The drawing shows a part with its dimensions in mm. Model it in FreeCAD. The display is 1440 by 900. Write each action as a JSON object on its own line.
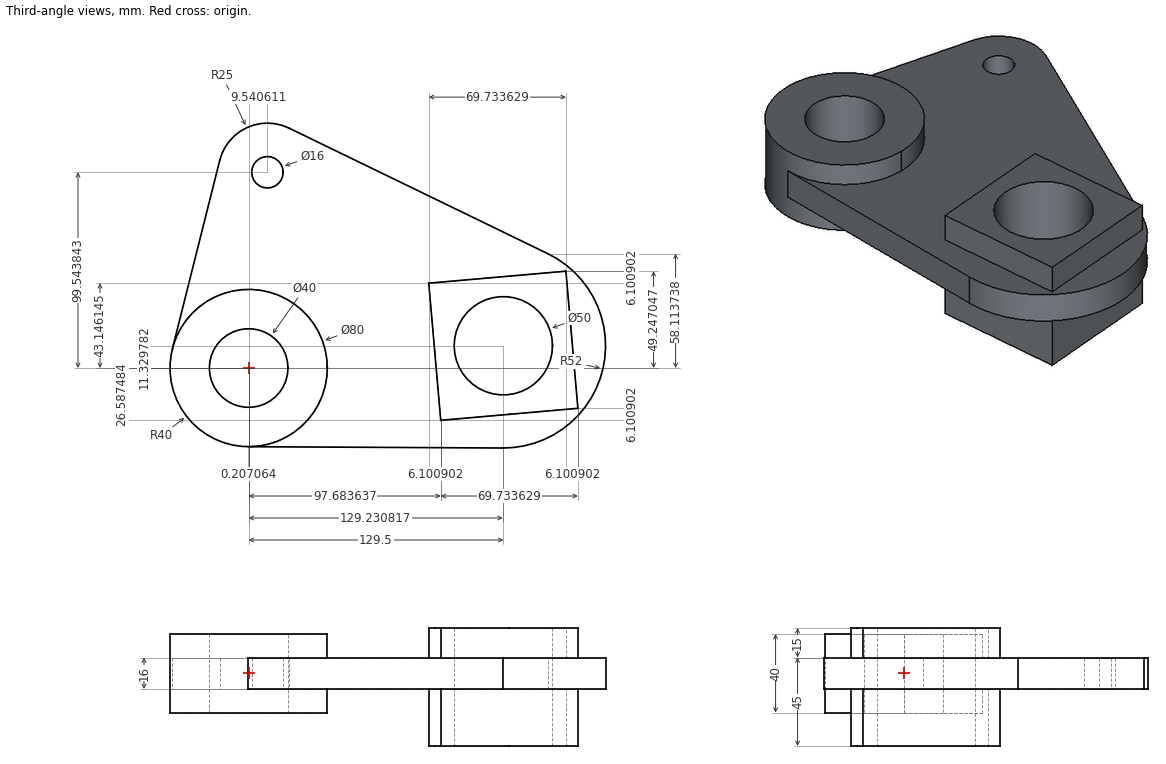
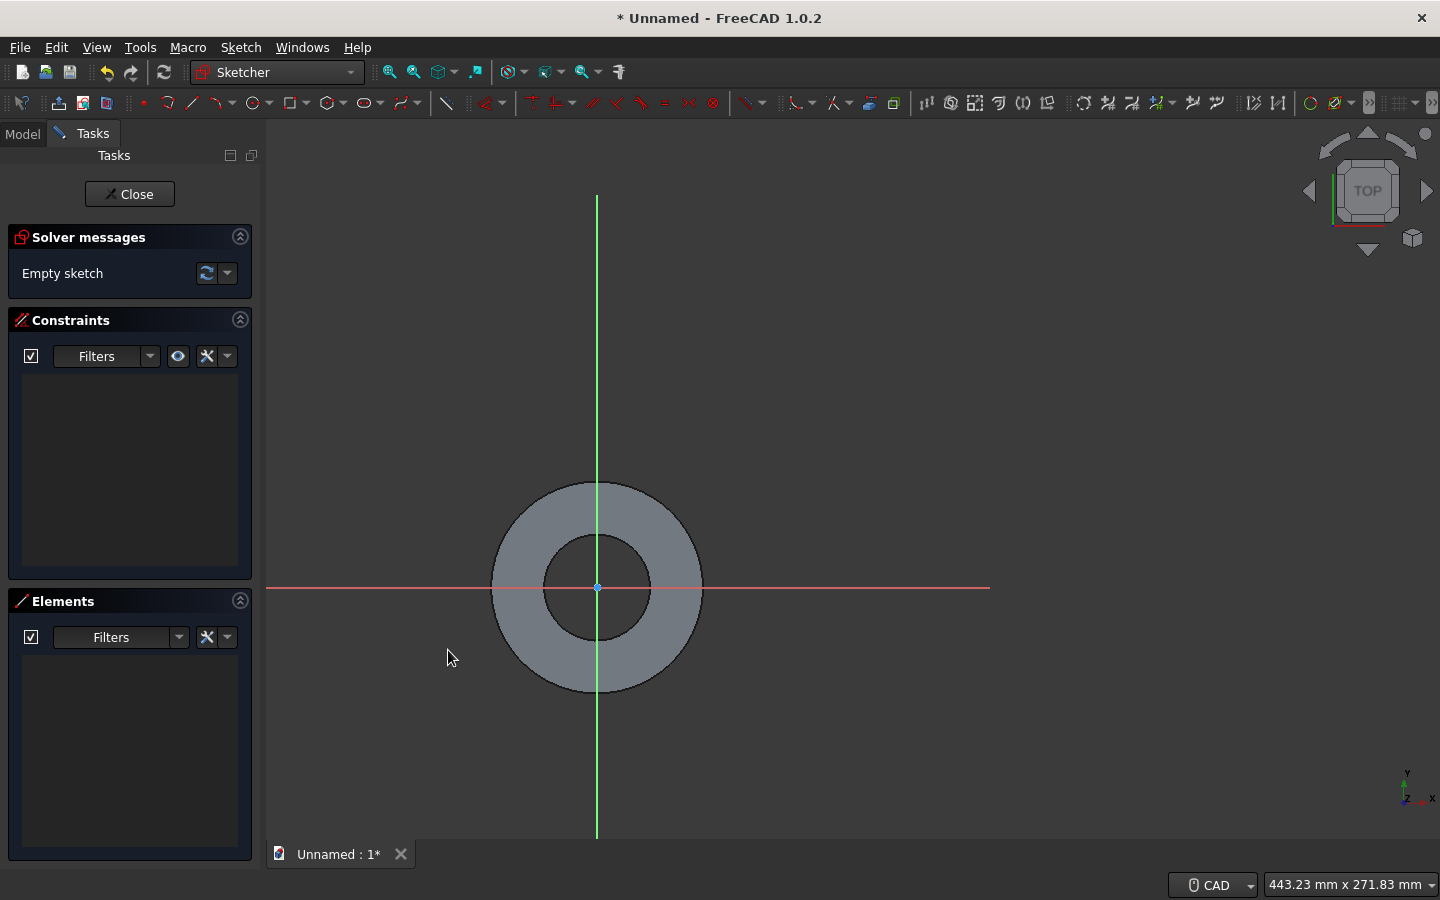
{"action": "key", "text": "g l"}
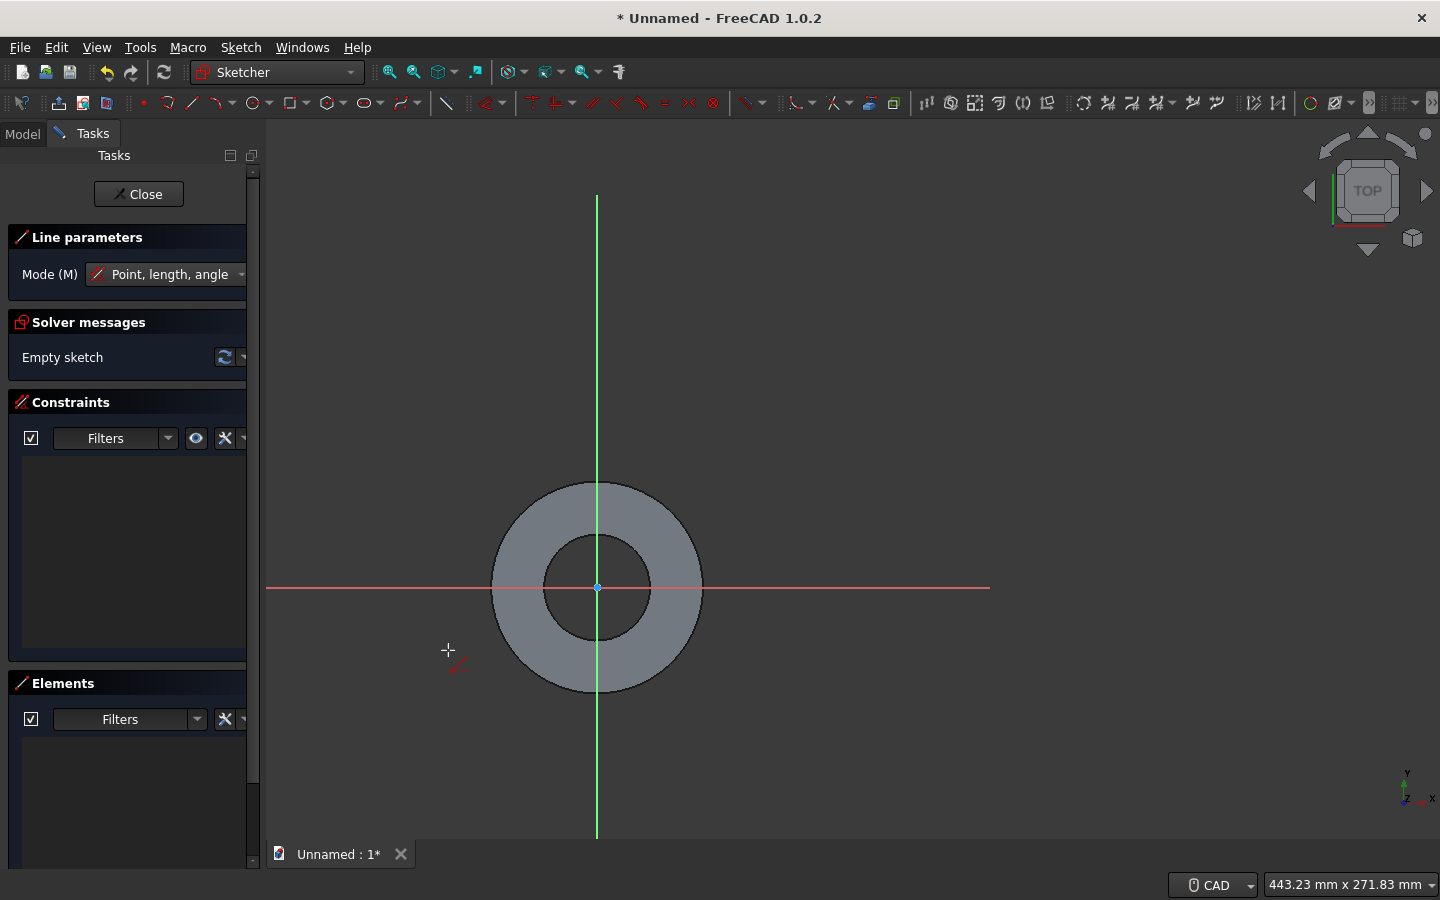
{"action": "scroll", "coordinate": [597, 694], "scroll_direction": "up", "scroll_amount": 17}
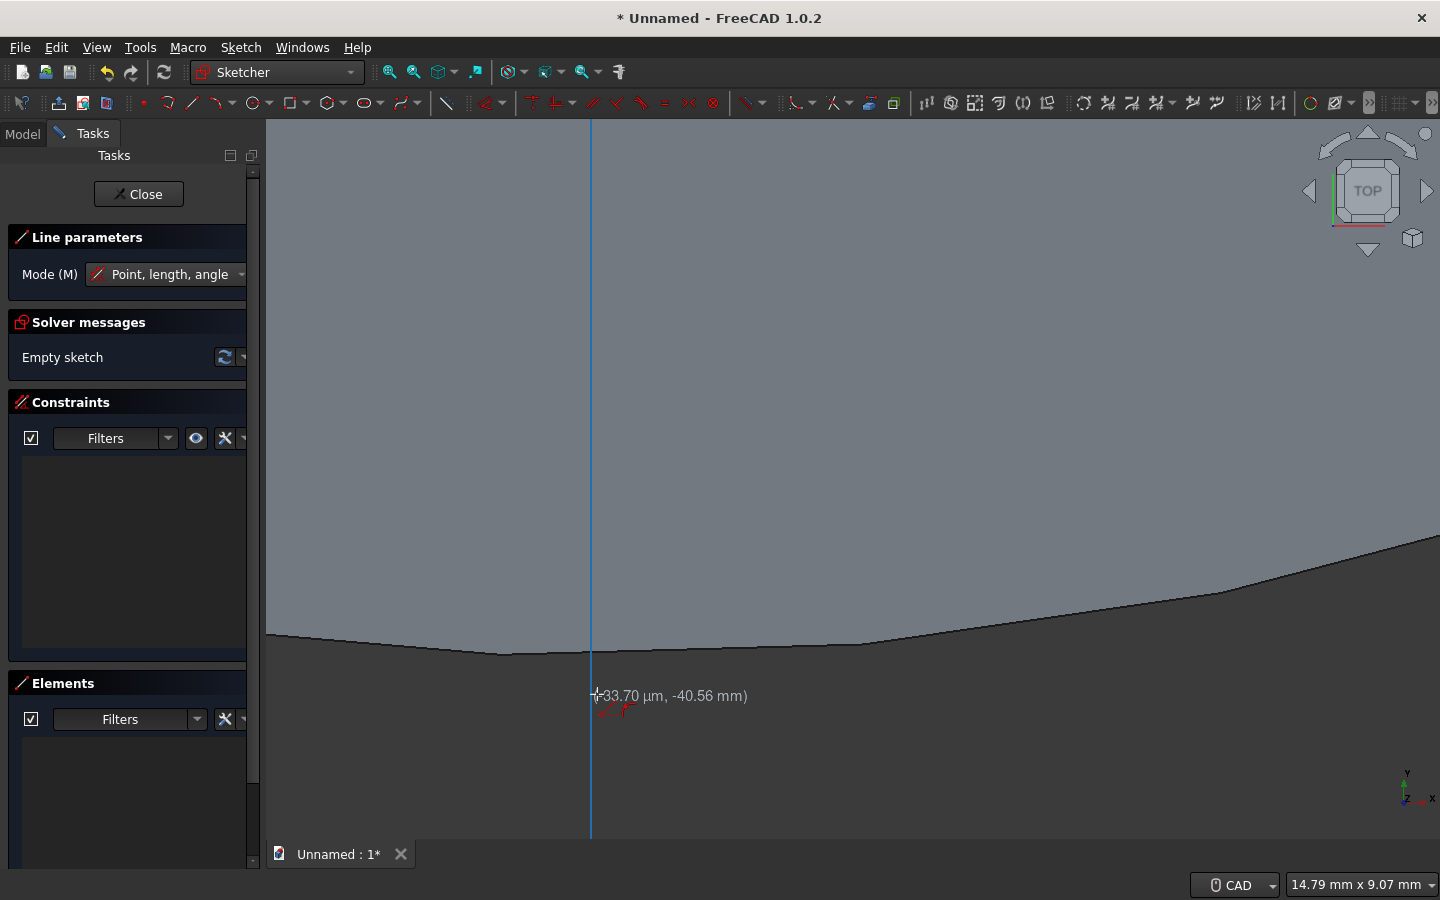
{"action": "left_click", "coordinate": [575, 656]}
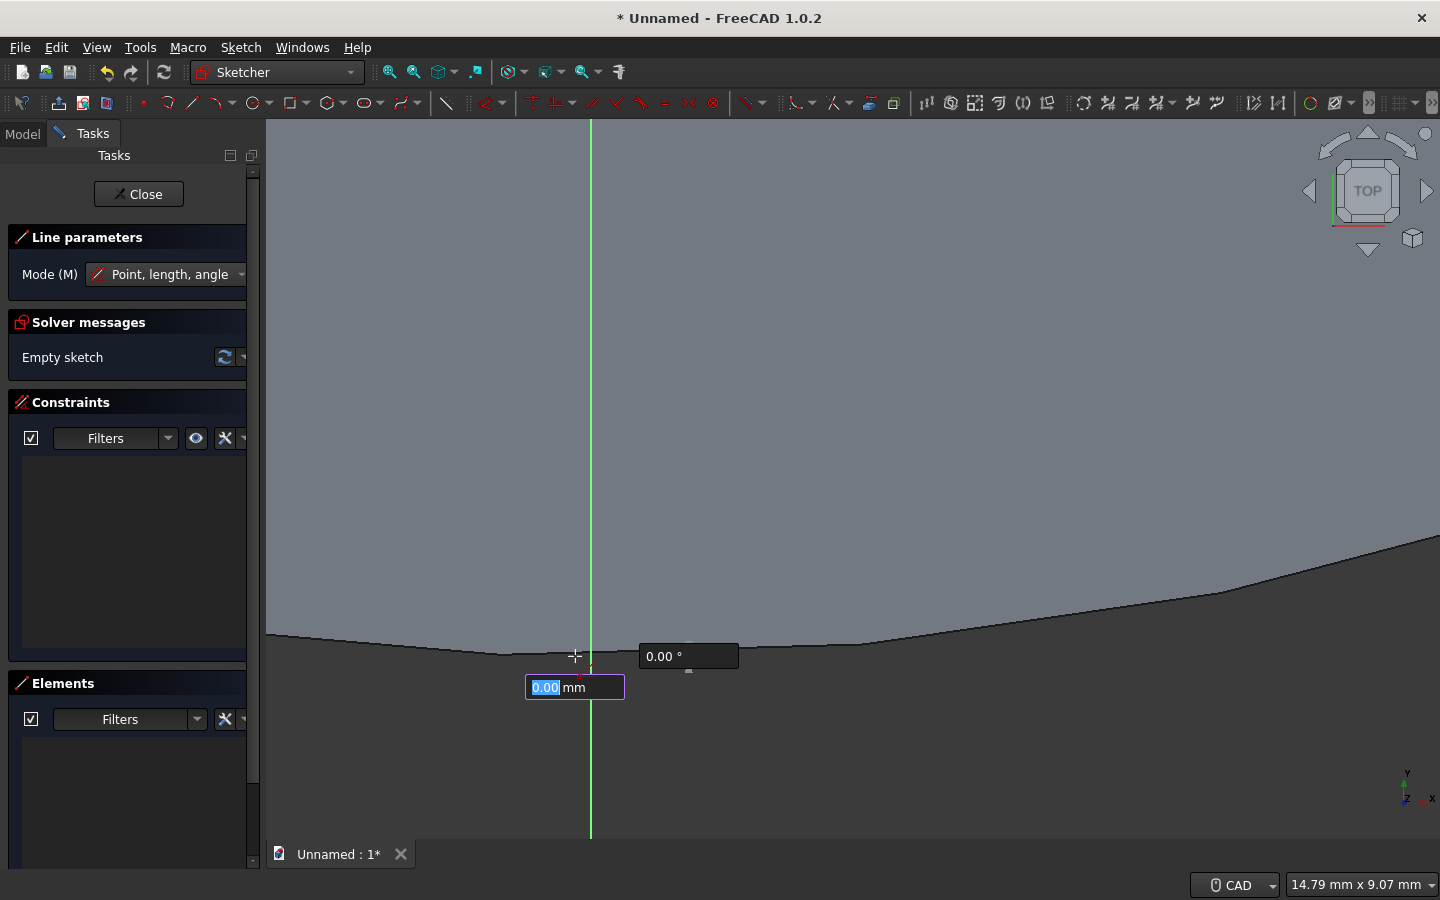
{"action": "scroll", "coordinate": [554, 744], "scroll_direction": "down", "scroll_amount": 16}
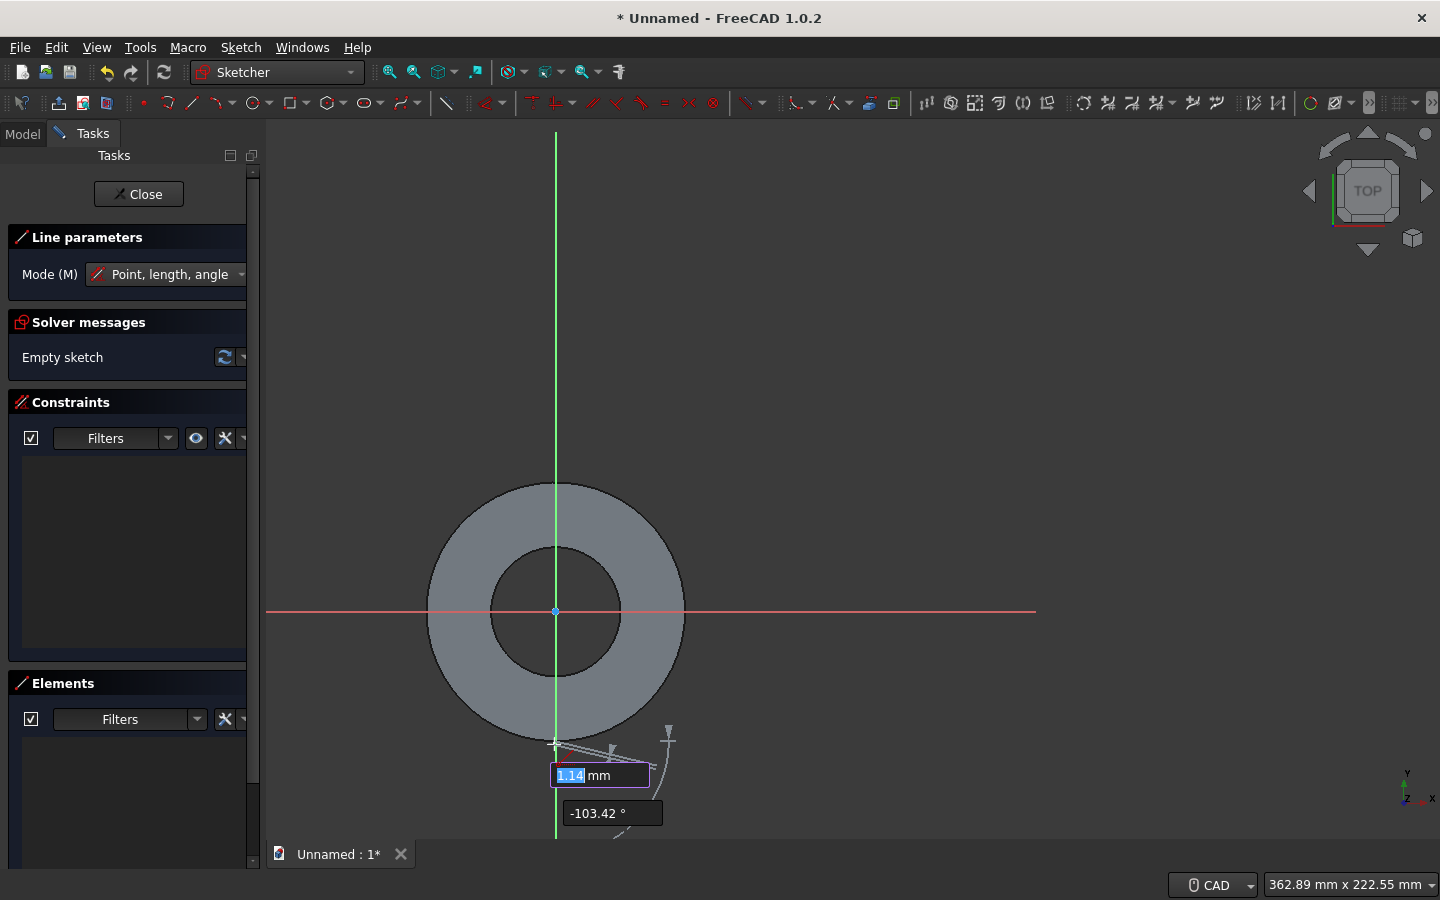
{"action": "left_click", "coordinate": [974, 762]}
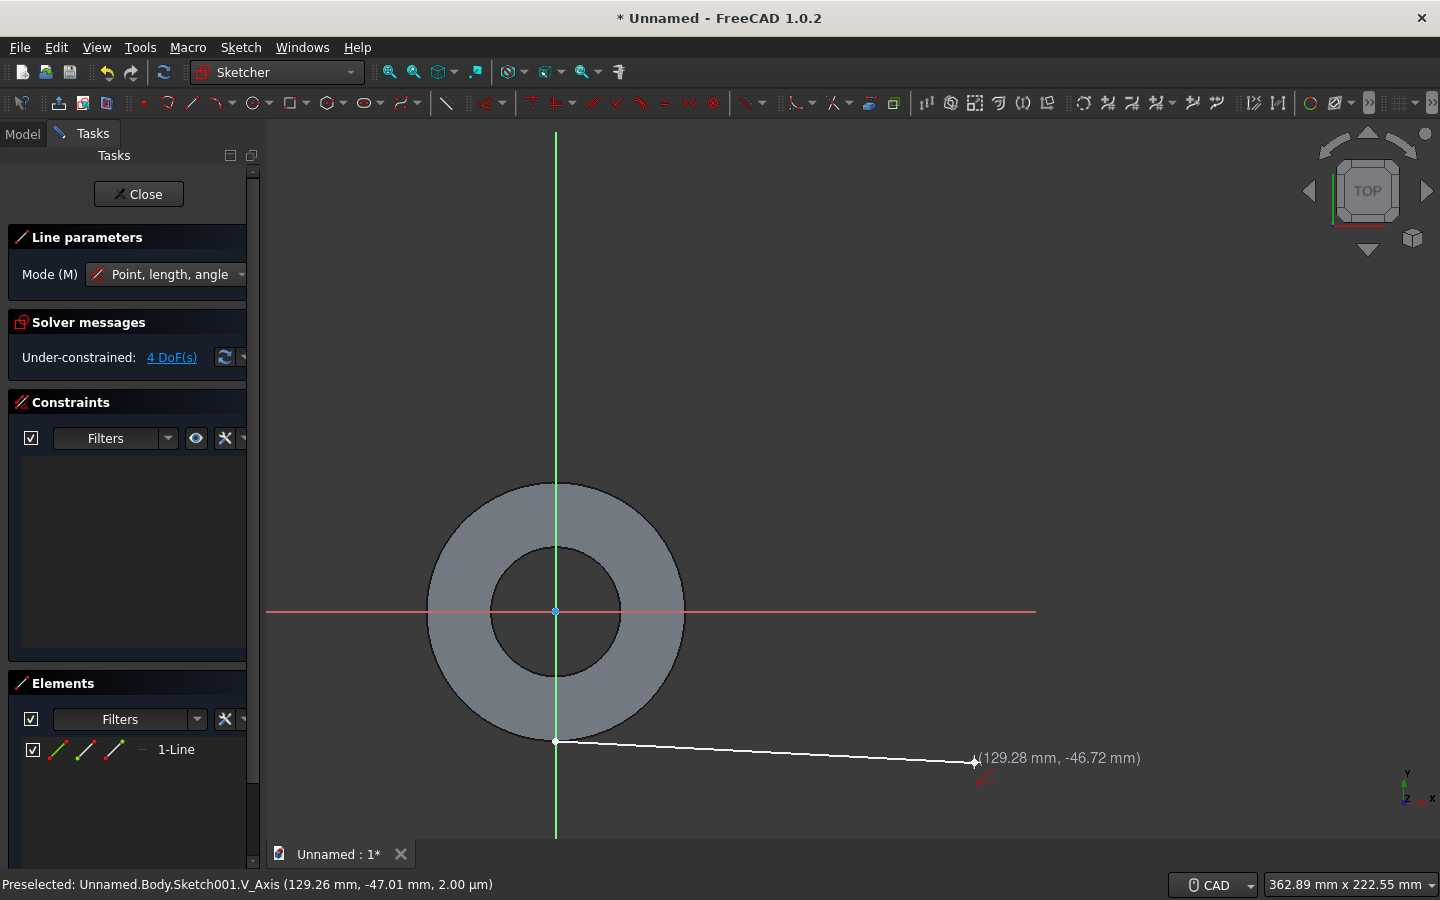
{"action": "left_click", "coordinate": [1048, 424]}
{"action": "left_click", "coordinate": [622, 217]}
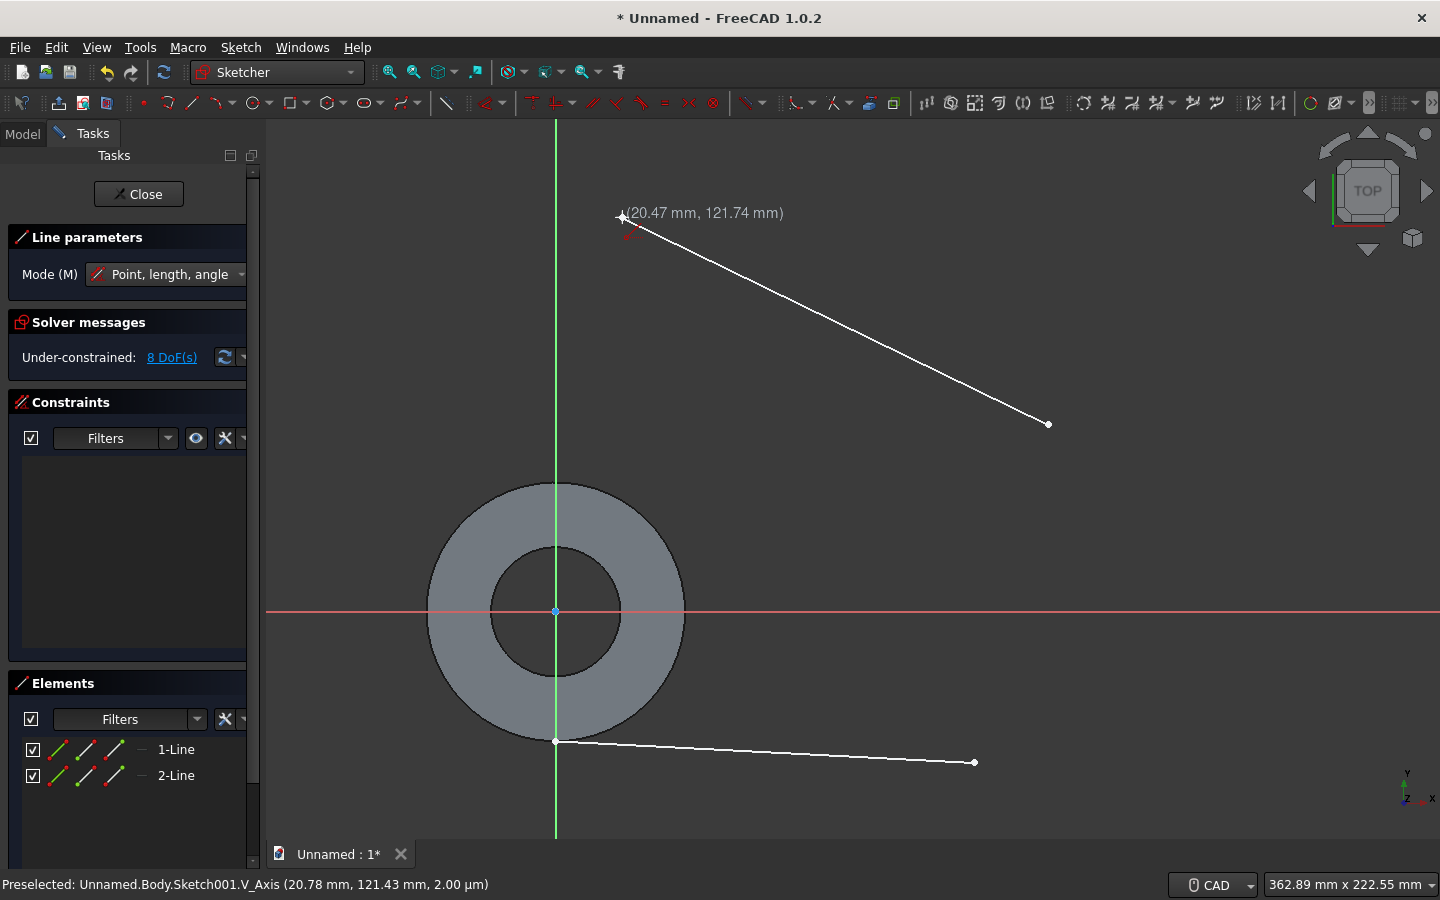
{"action": "left_click", "coordinate": [508, 270]}
{"action": "left_click", "coordinate": [430, 580]}